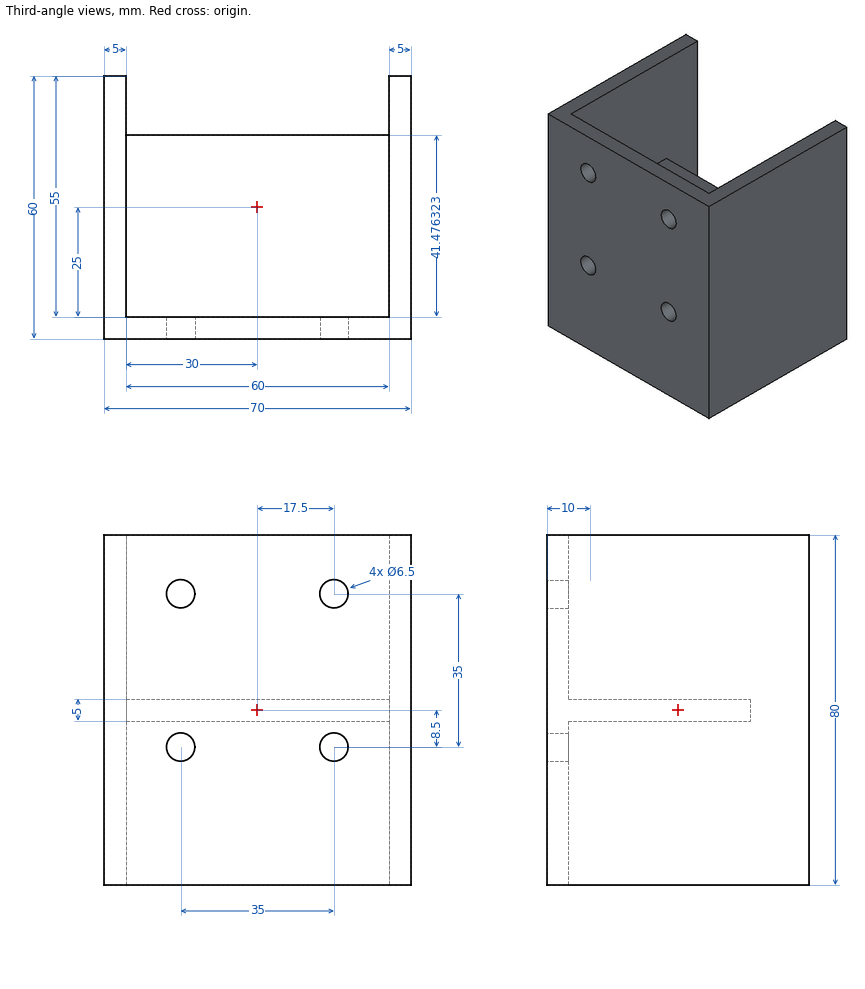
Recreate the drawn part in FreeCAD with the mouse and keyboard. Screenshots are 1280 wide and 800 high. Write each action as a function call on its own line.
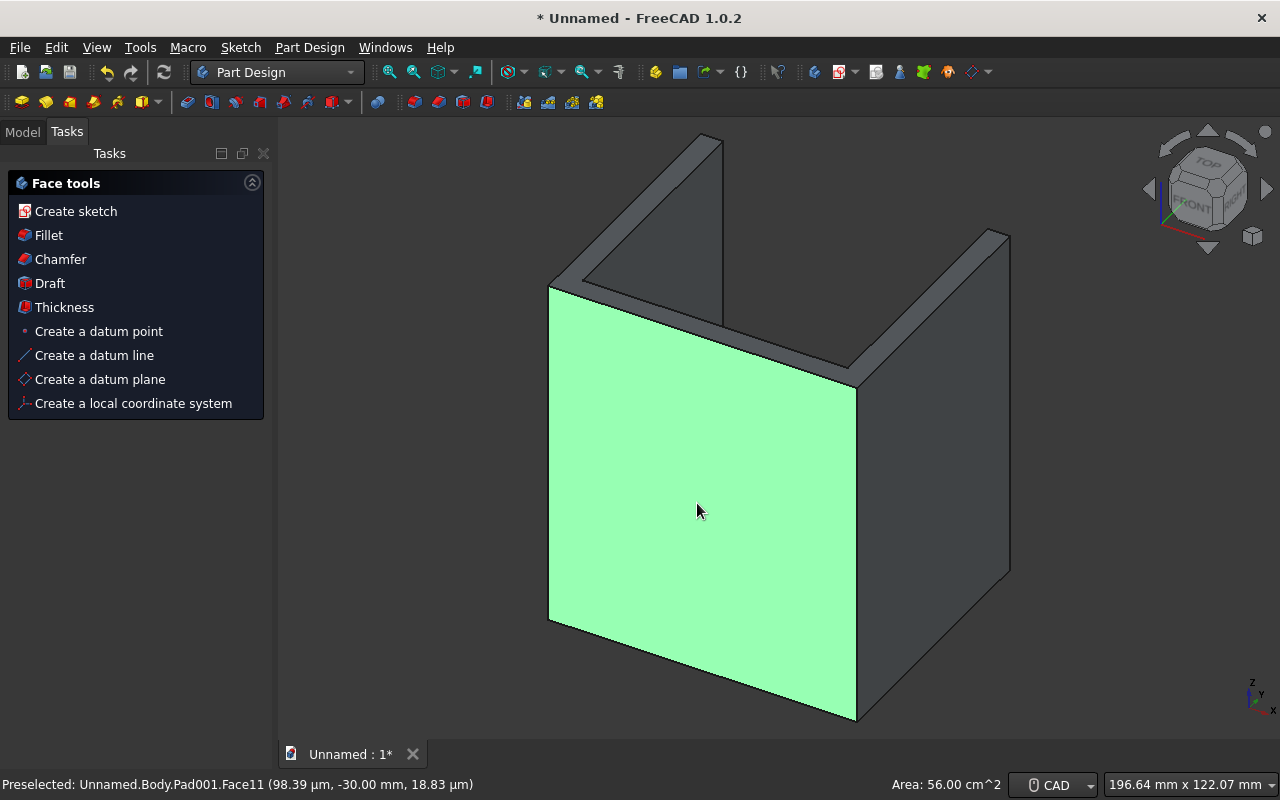
click(840, 72)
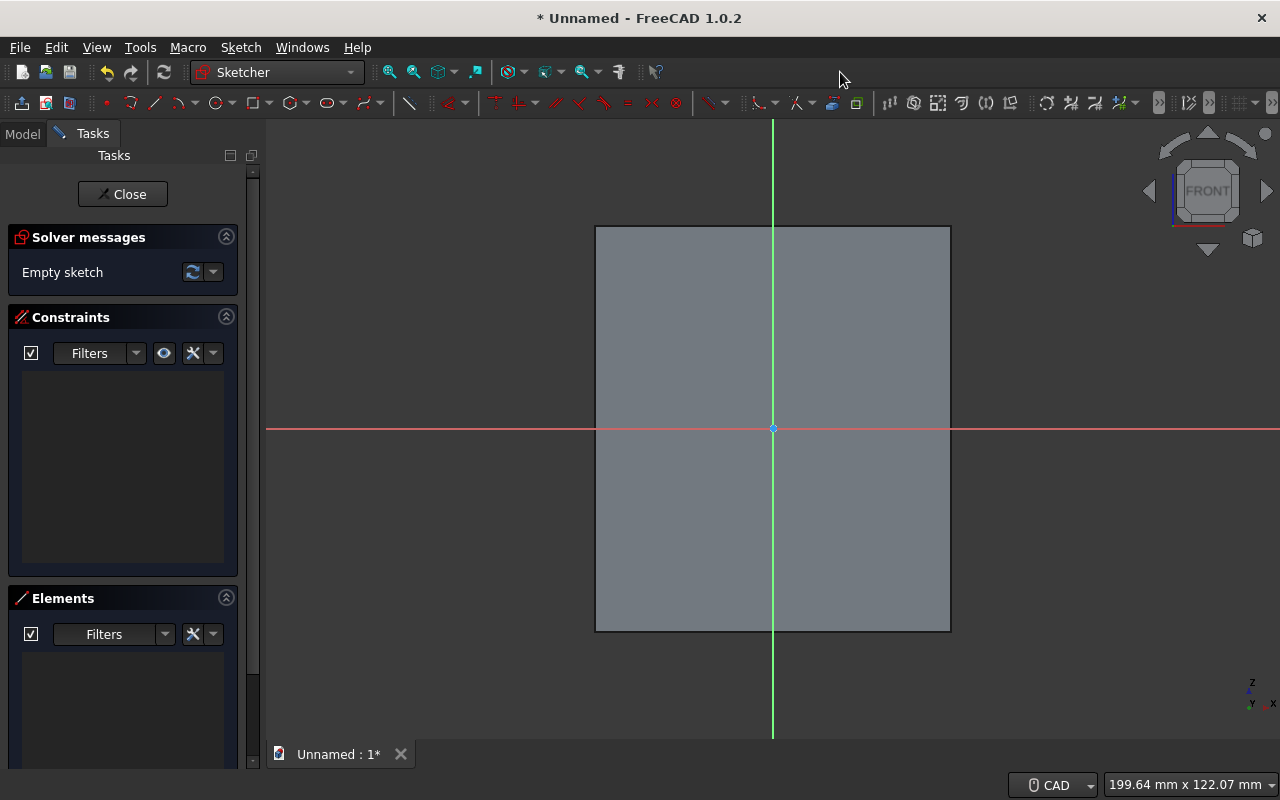
scroll(856, 328, up, 3)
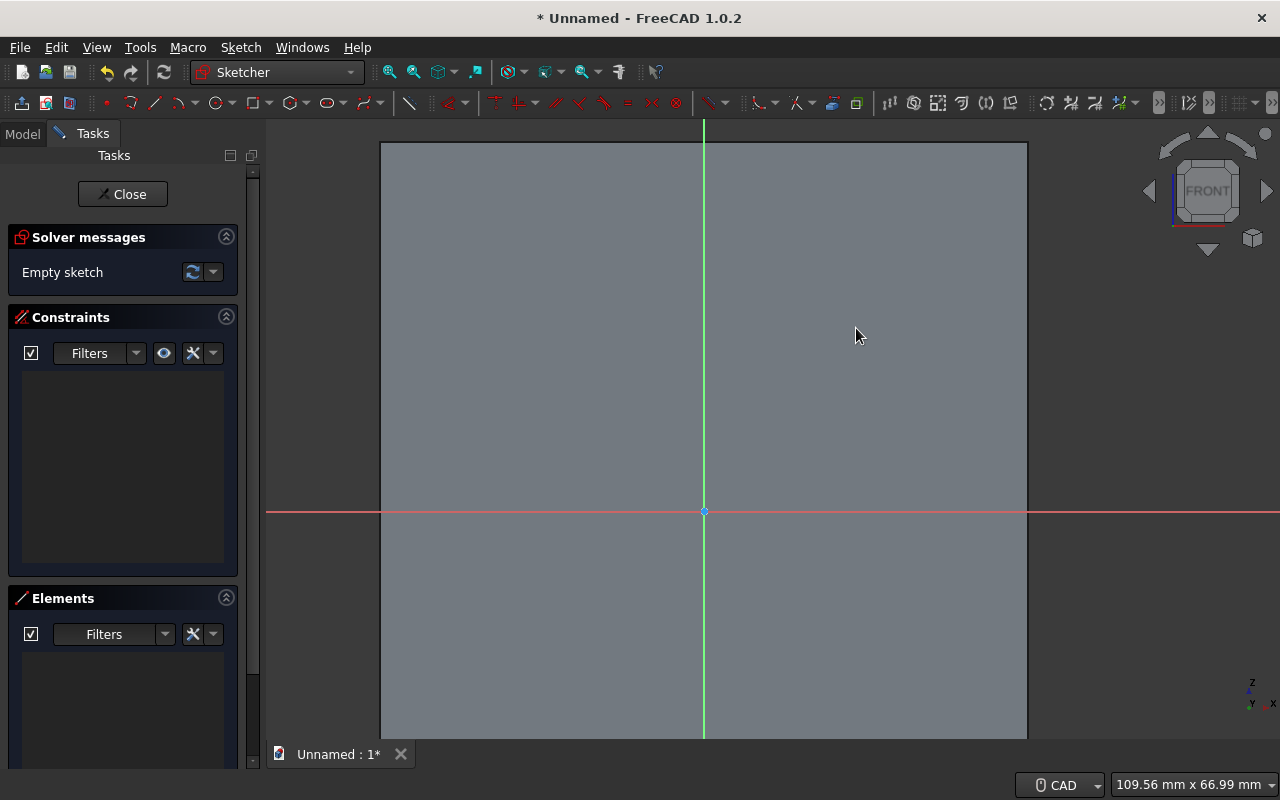
key(g)
key(c)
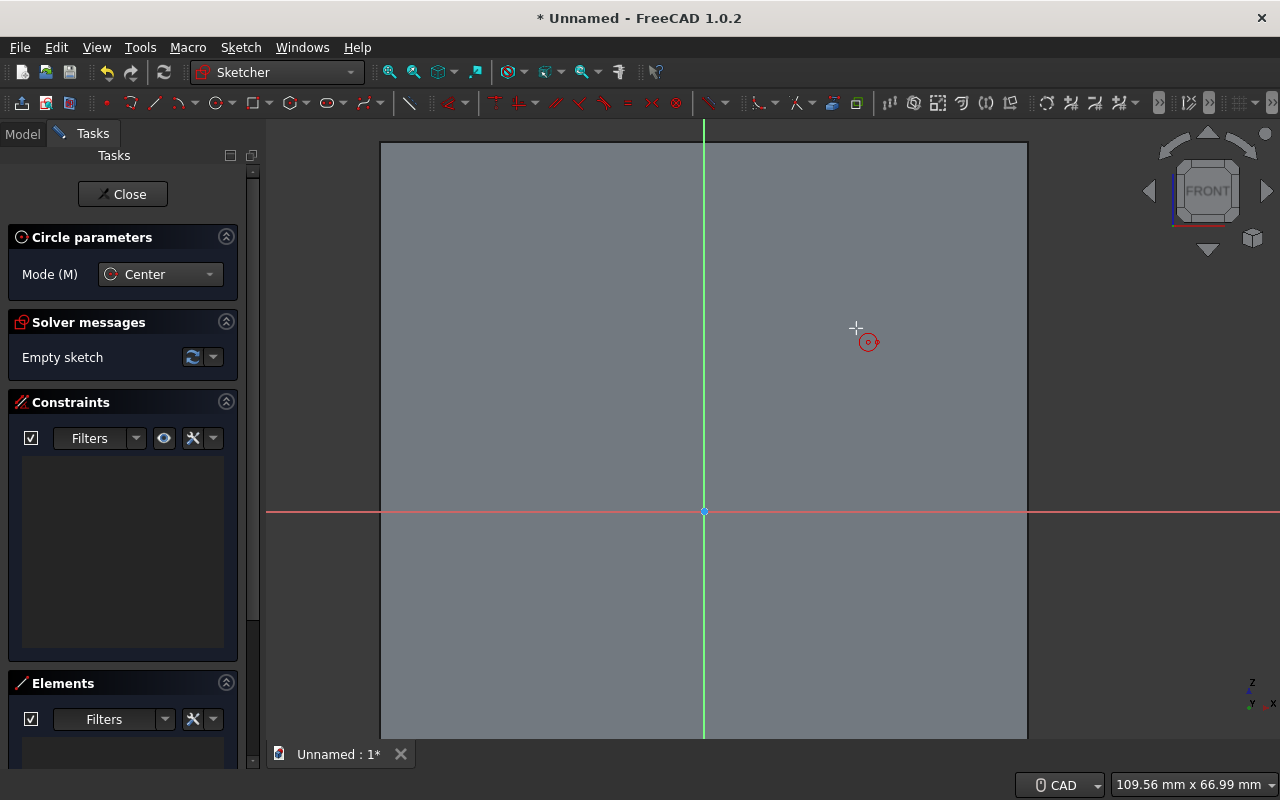
click(866, 266)
move(888, 245)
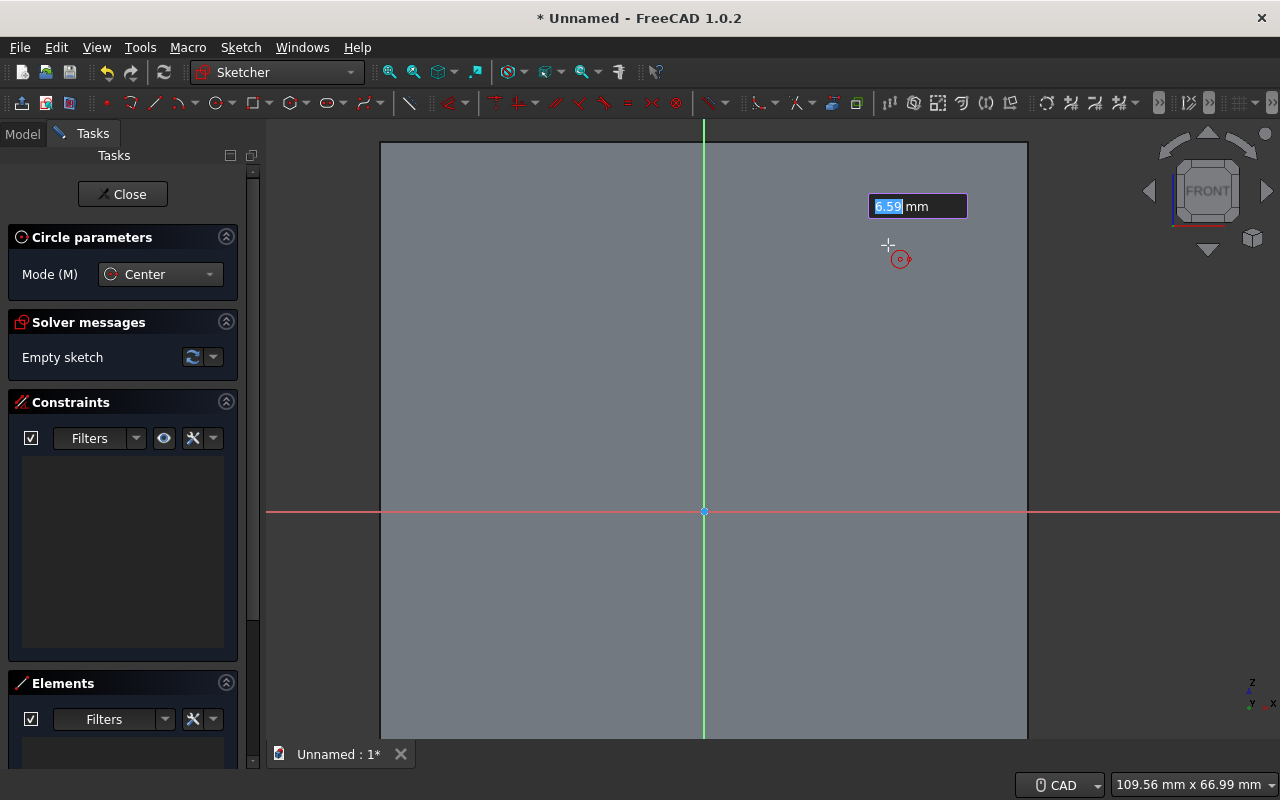
text(6.5)
key(Return)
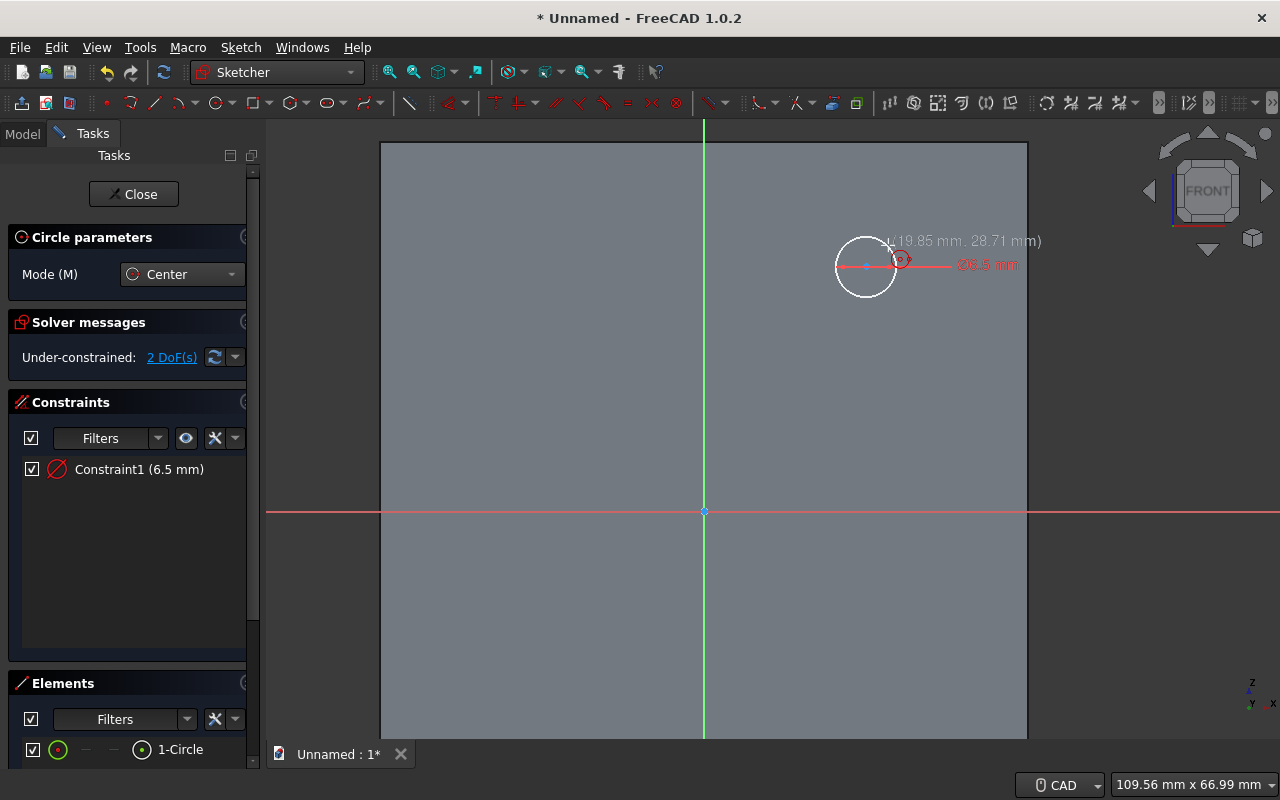
click(866, 590)
move(888, 569)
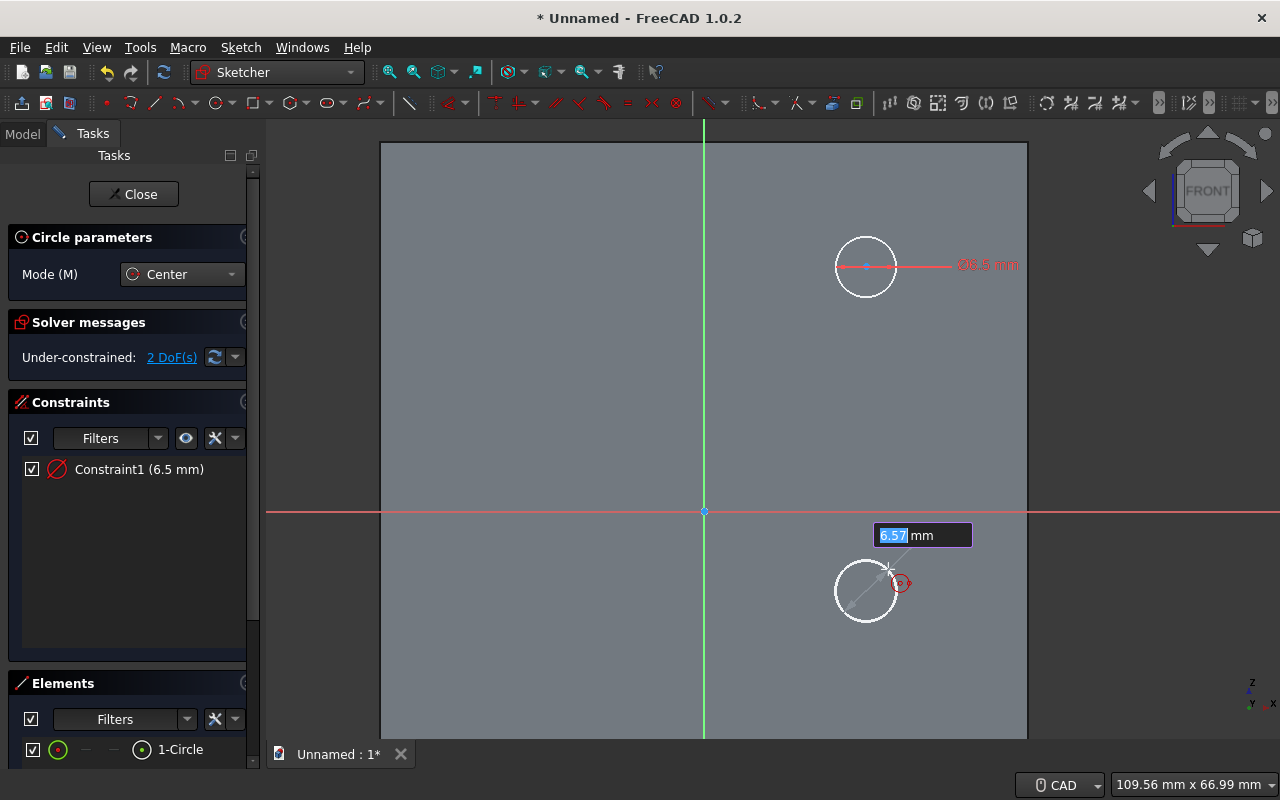
text(6.5)
key(Return)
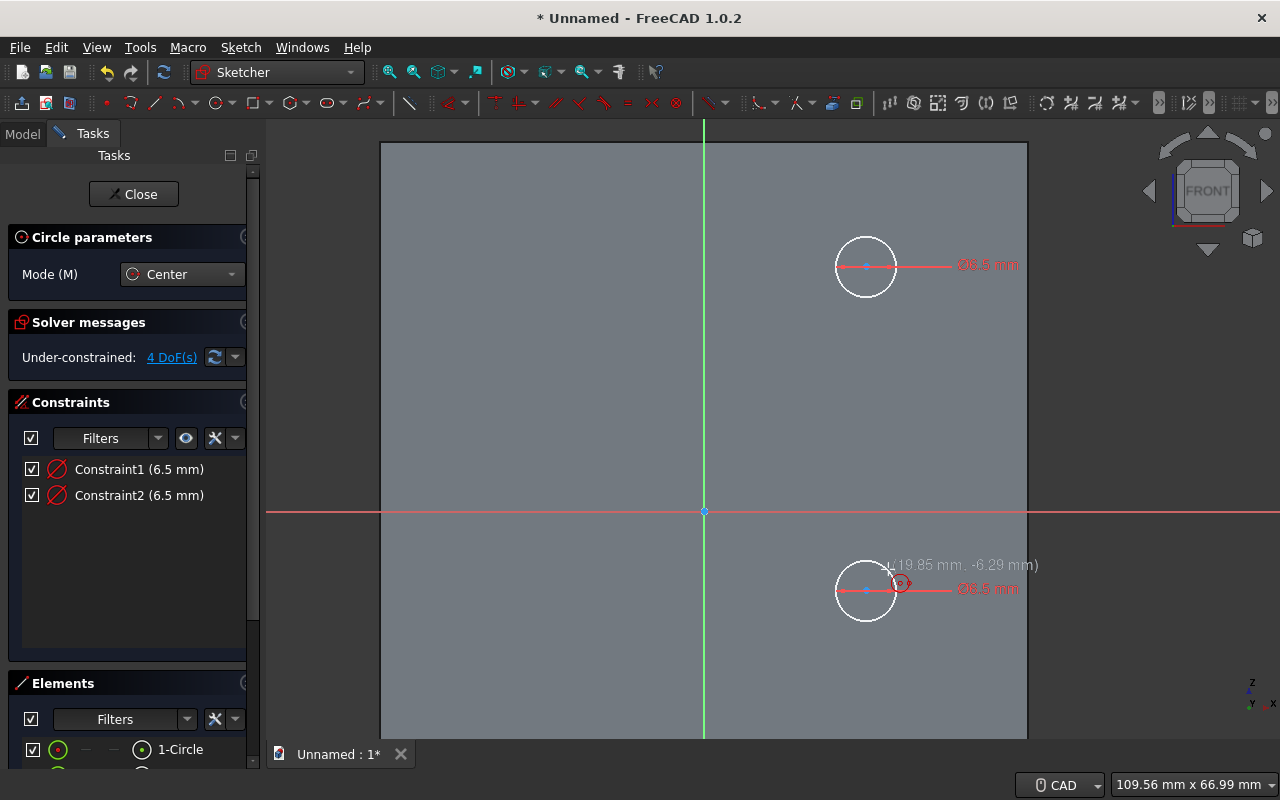
click(542, 590)
move(564, 569)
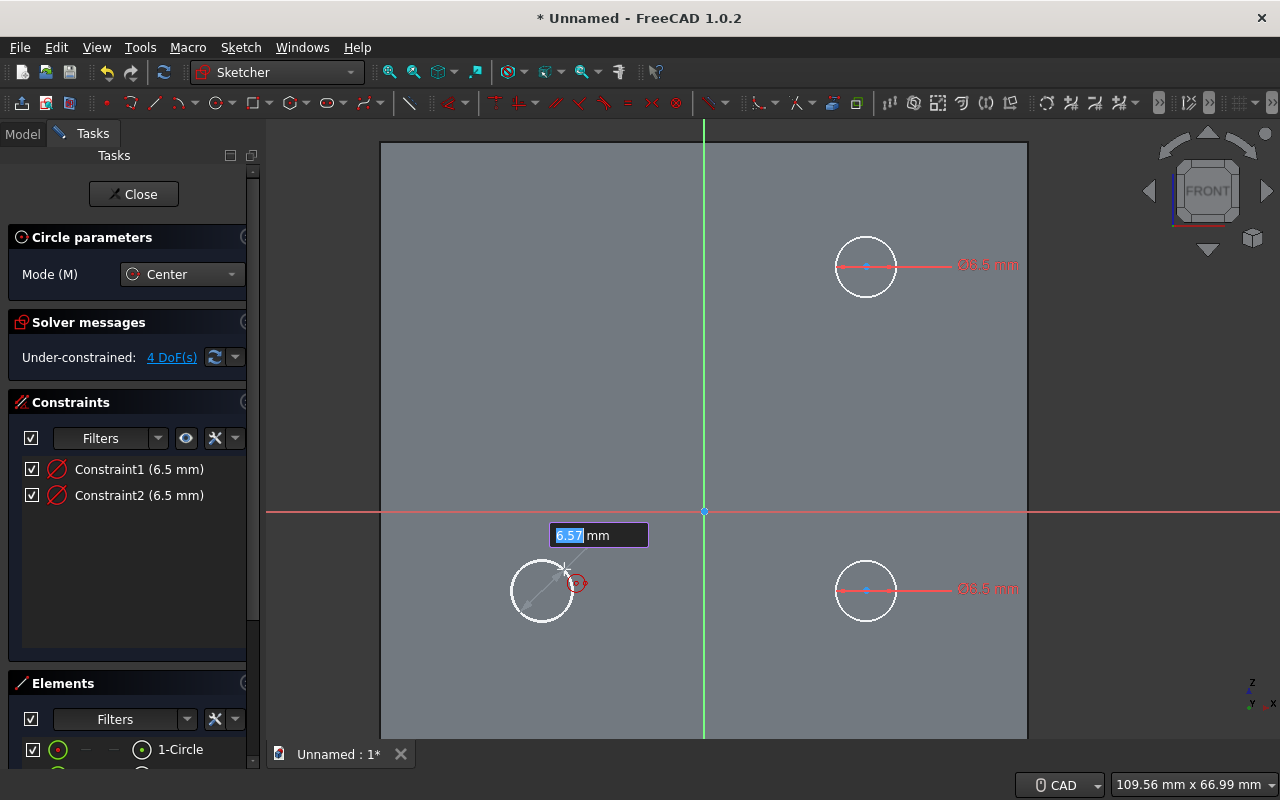
text(6.5)
key(Return)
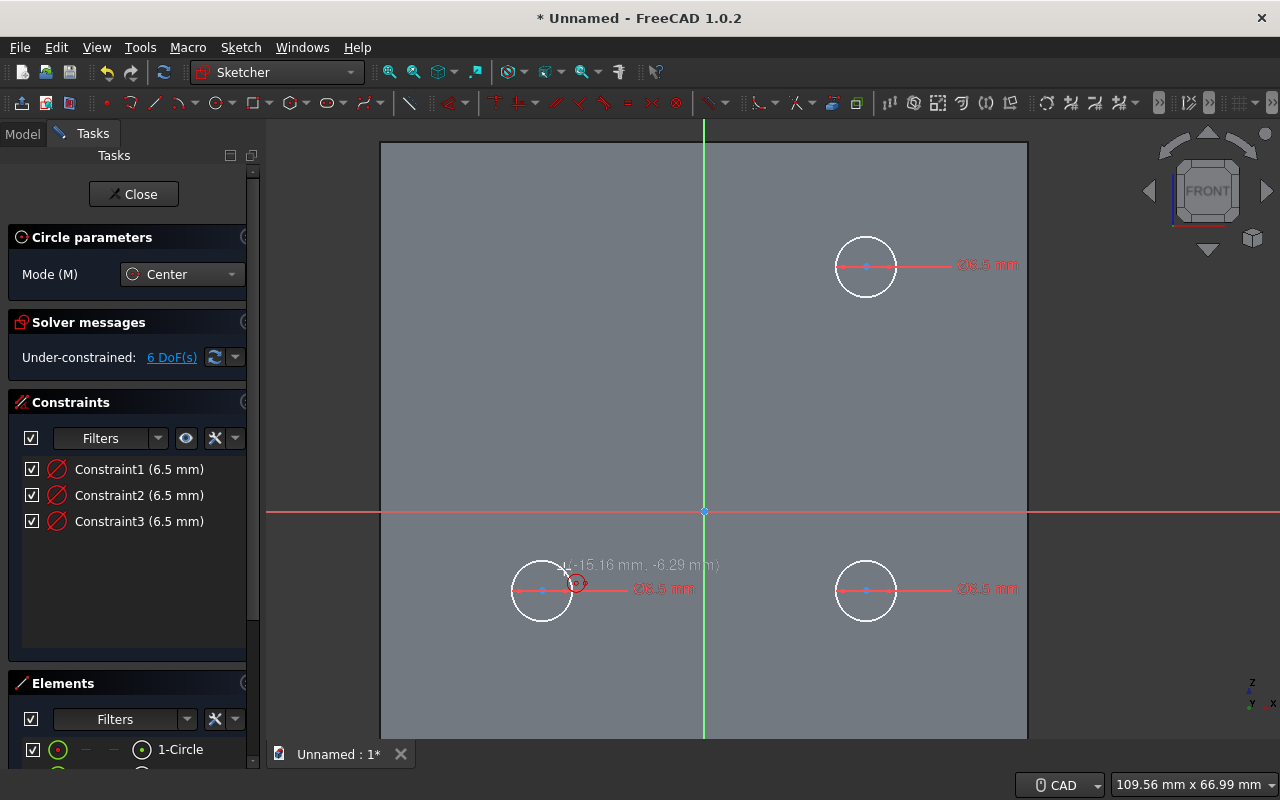
click(542, 266)
move(564, 245)